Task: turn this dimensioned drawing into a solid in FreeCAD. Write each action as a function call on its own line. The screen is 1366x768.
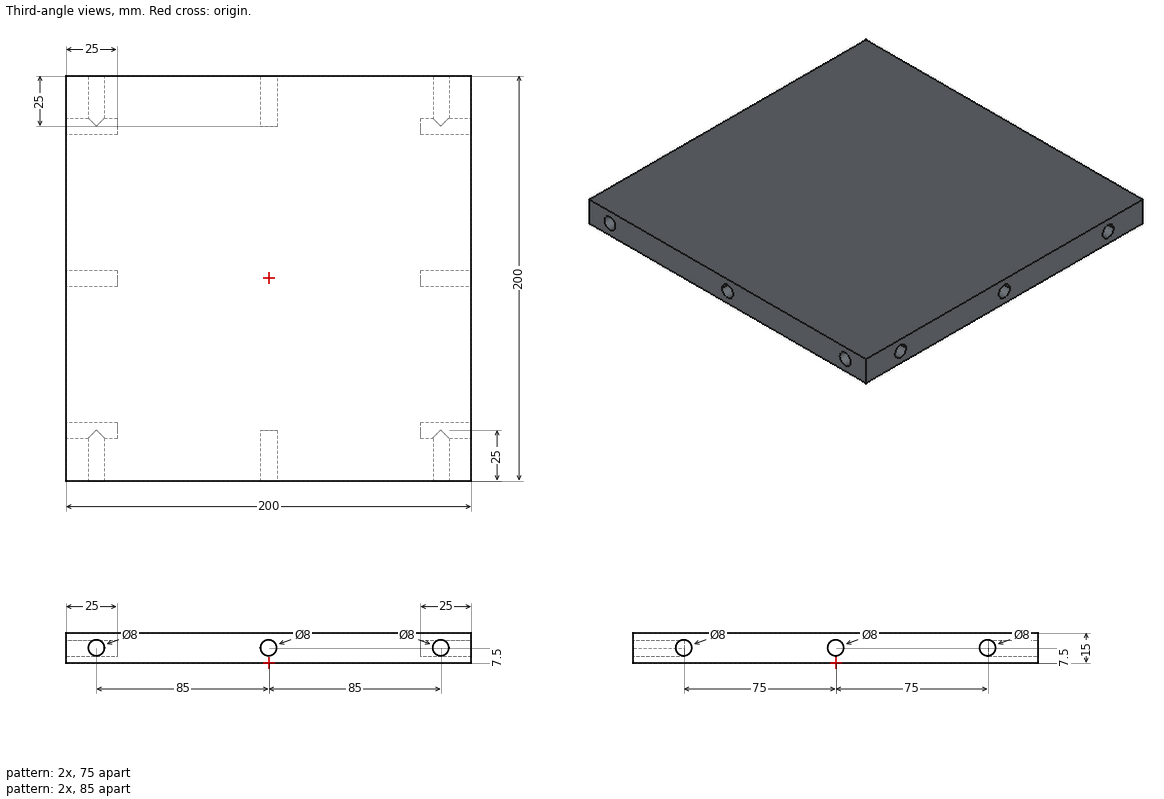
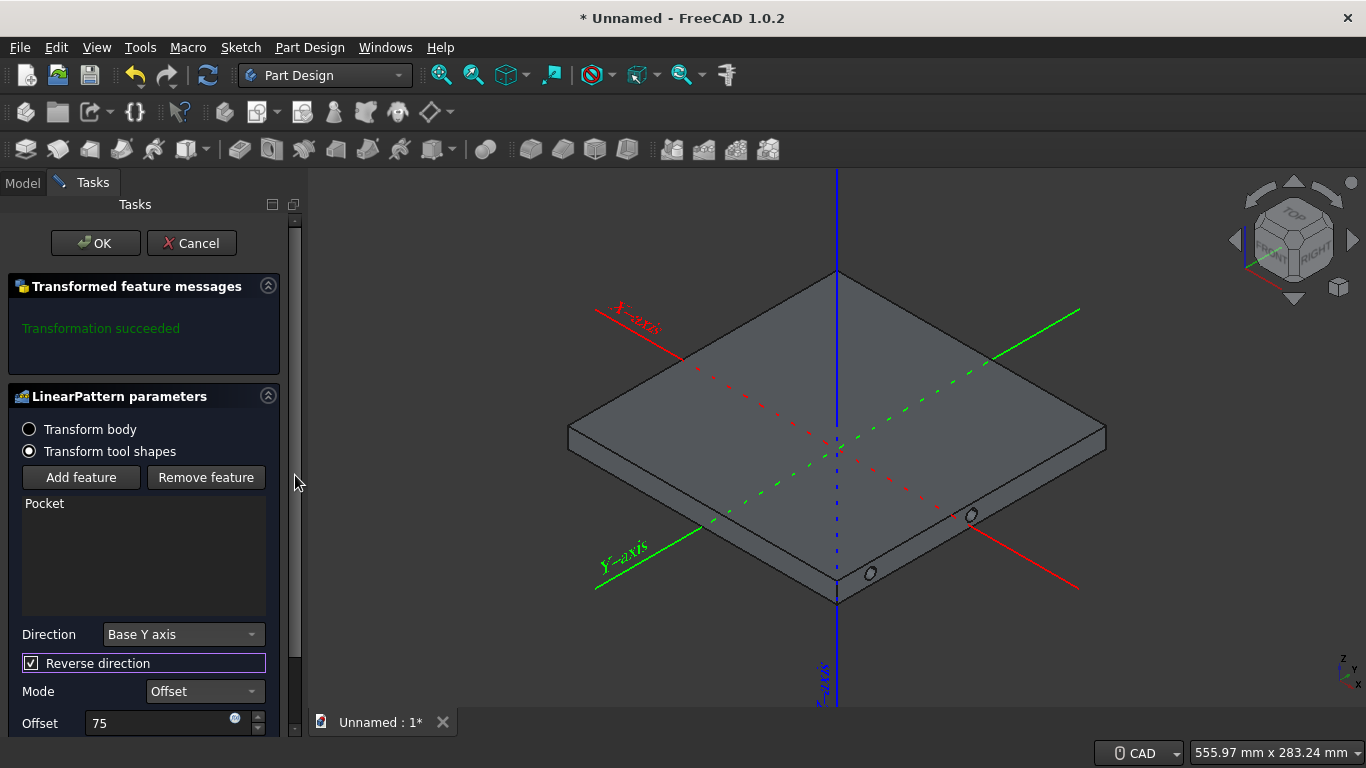
click(96, 243)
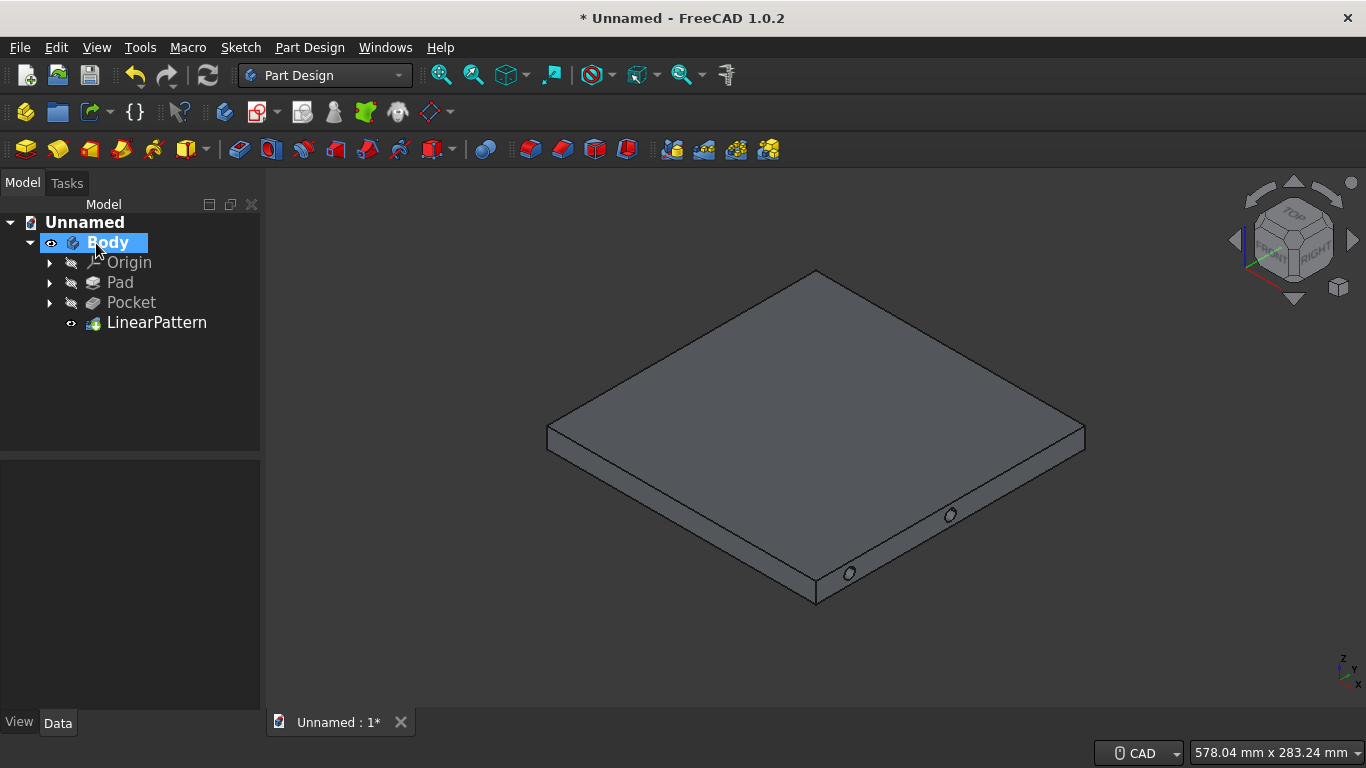
click(1066, 448)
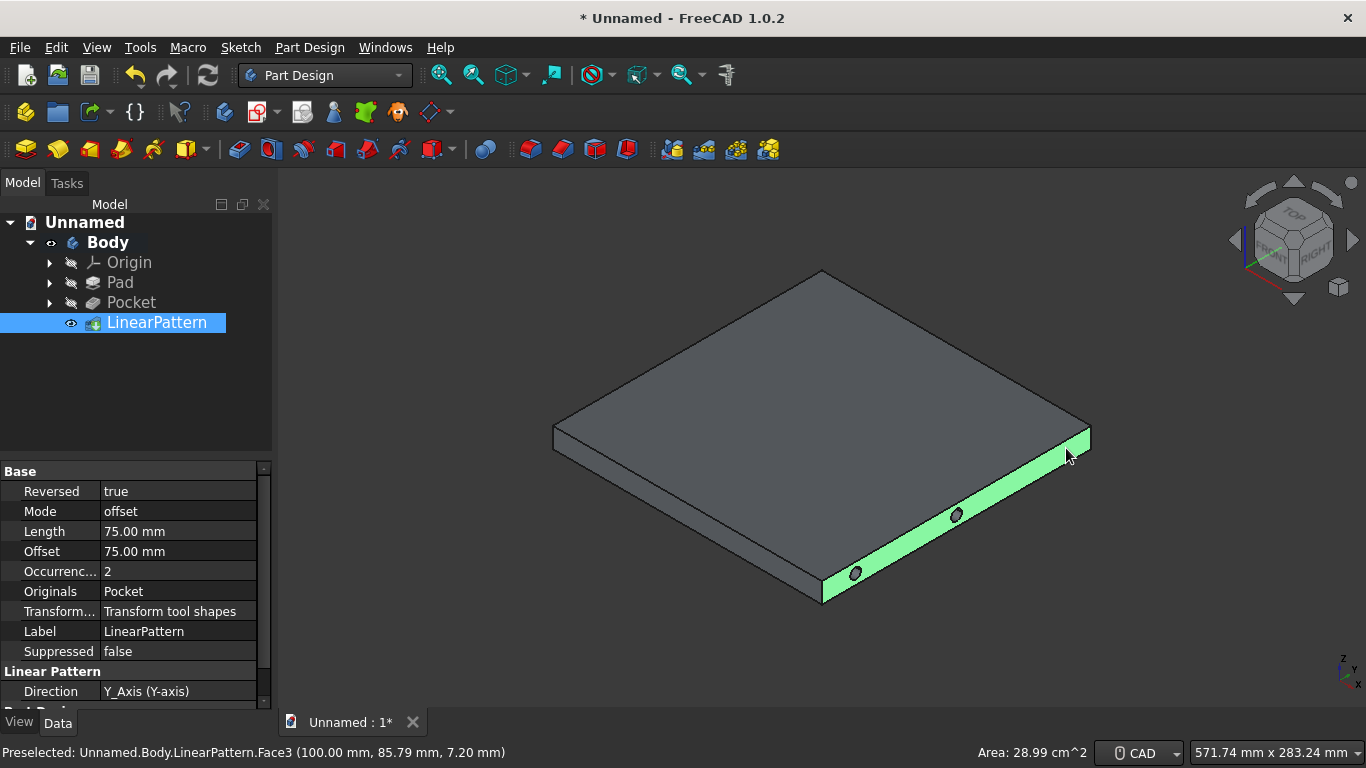
click(258, 112)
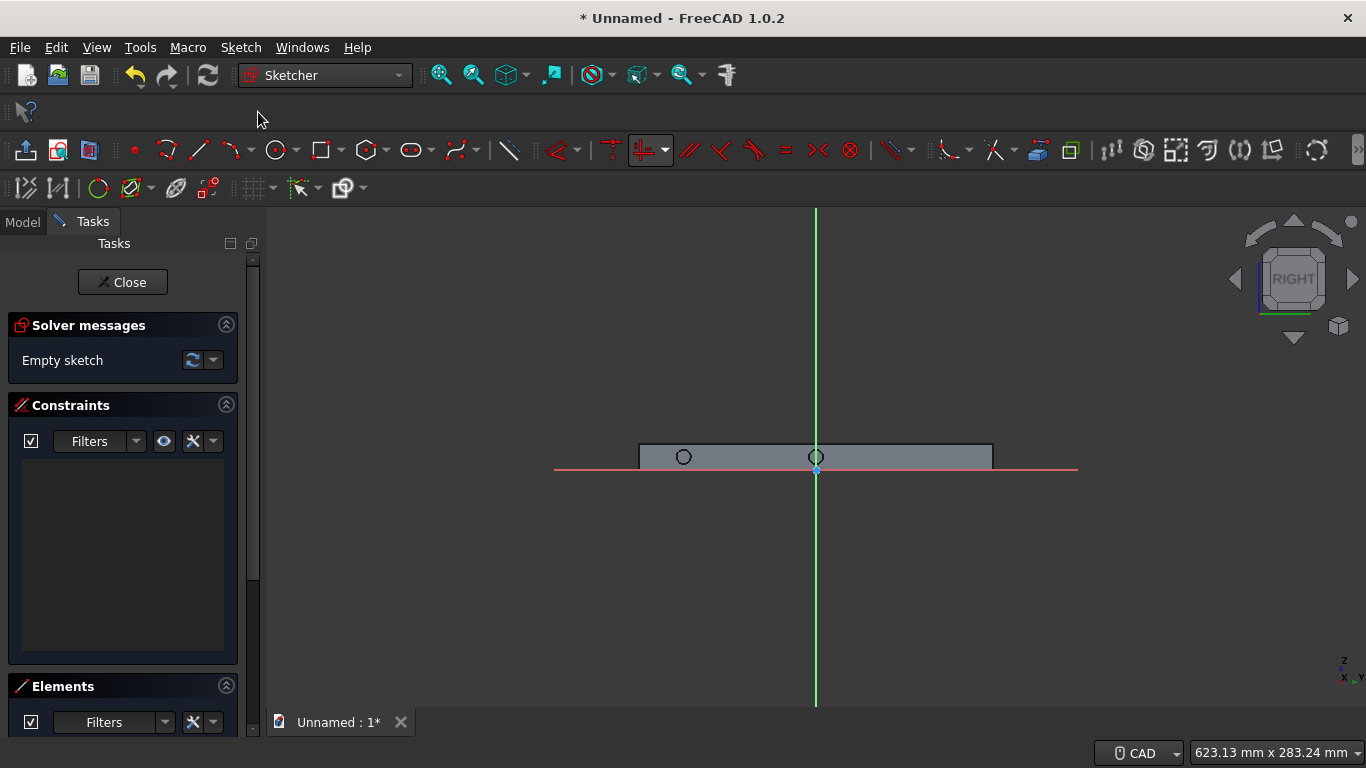
scroll(959, 457, up, 15)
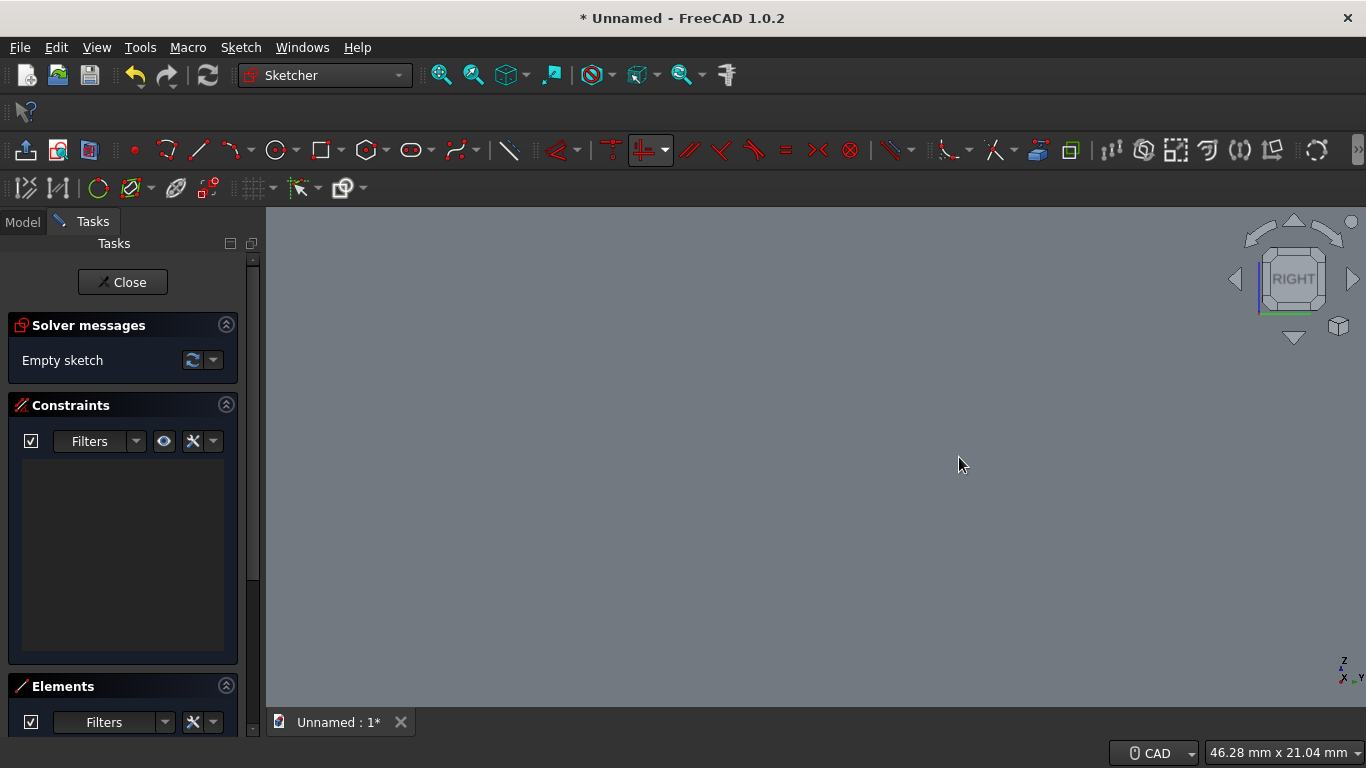
click(276, 150)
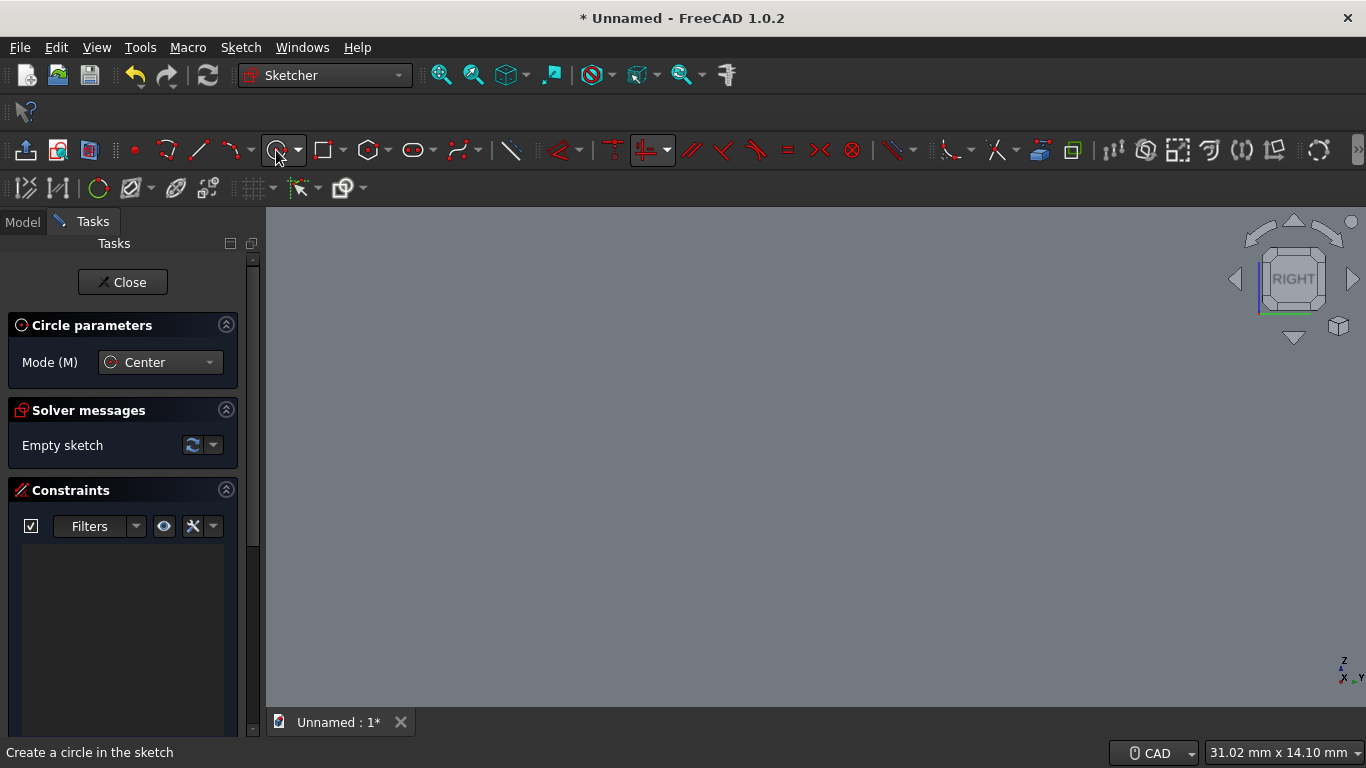
click(734, 447)
move(834, 347)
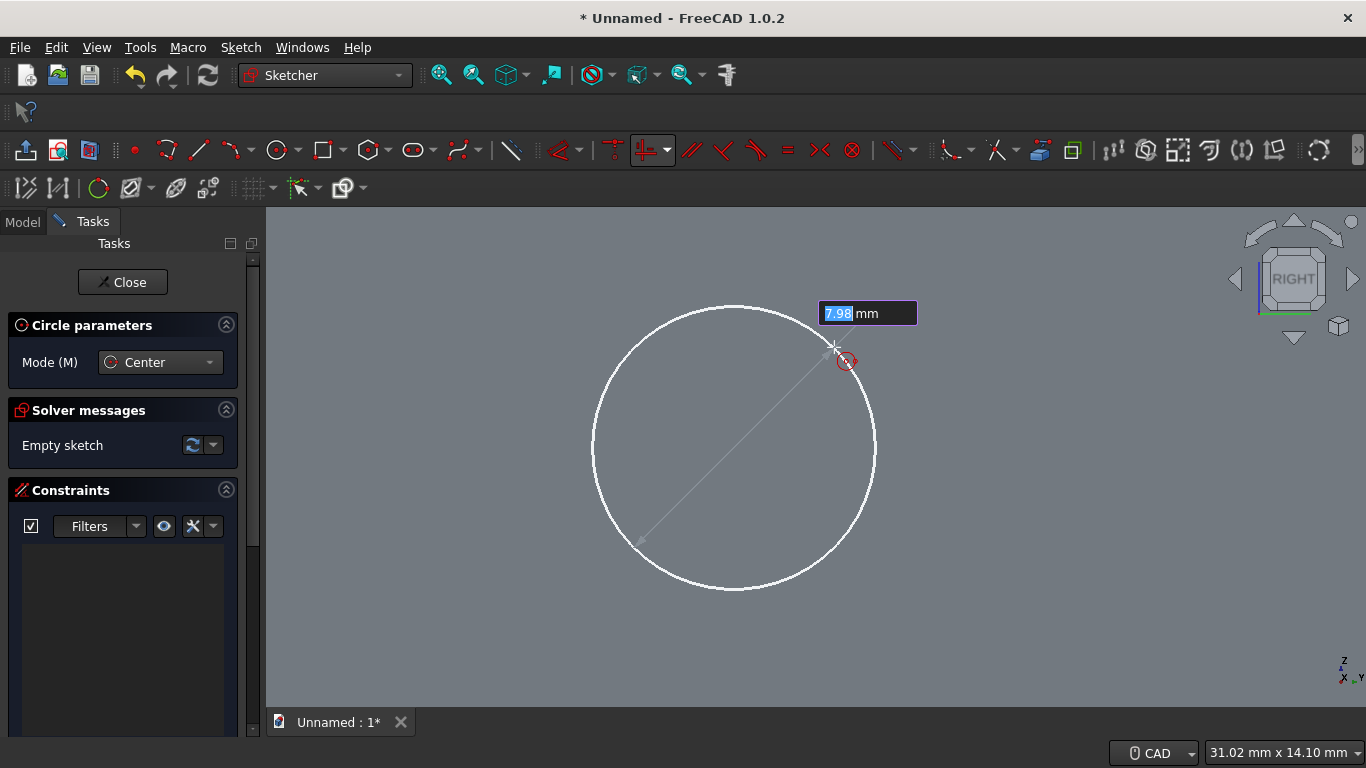
text(8)
key(Return)
key(Escape)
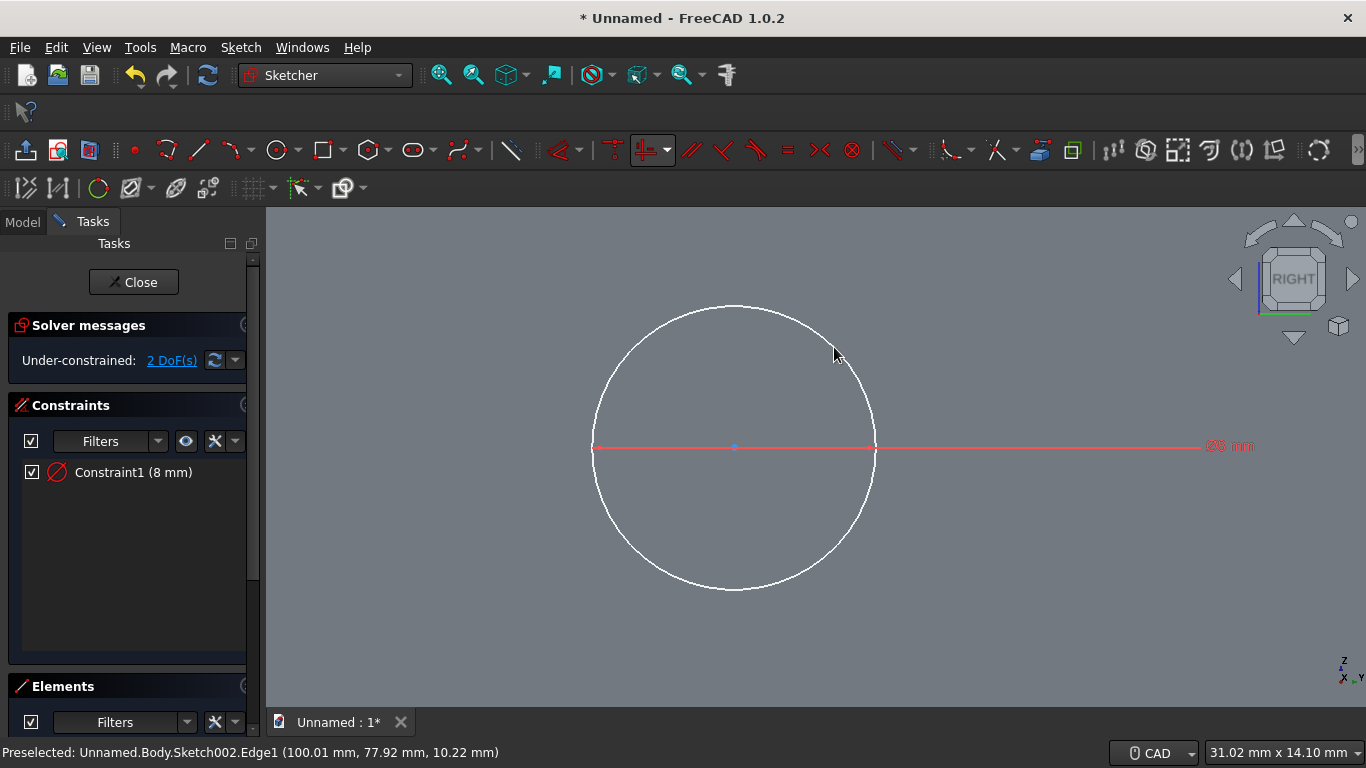
click(558, 150)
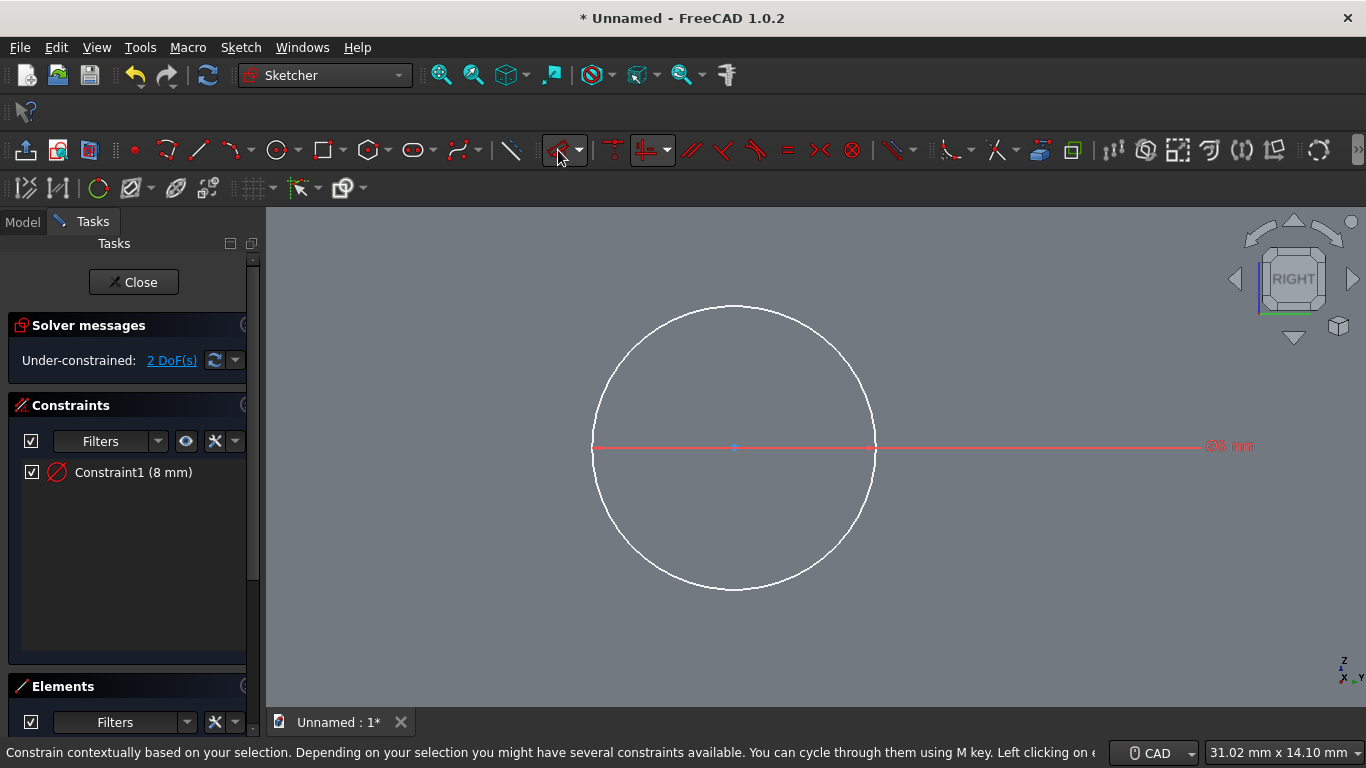
click(734, 448)
click(514, 414)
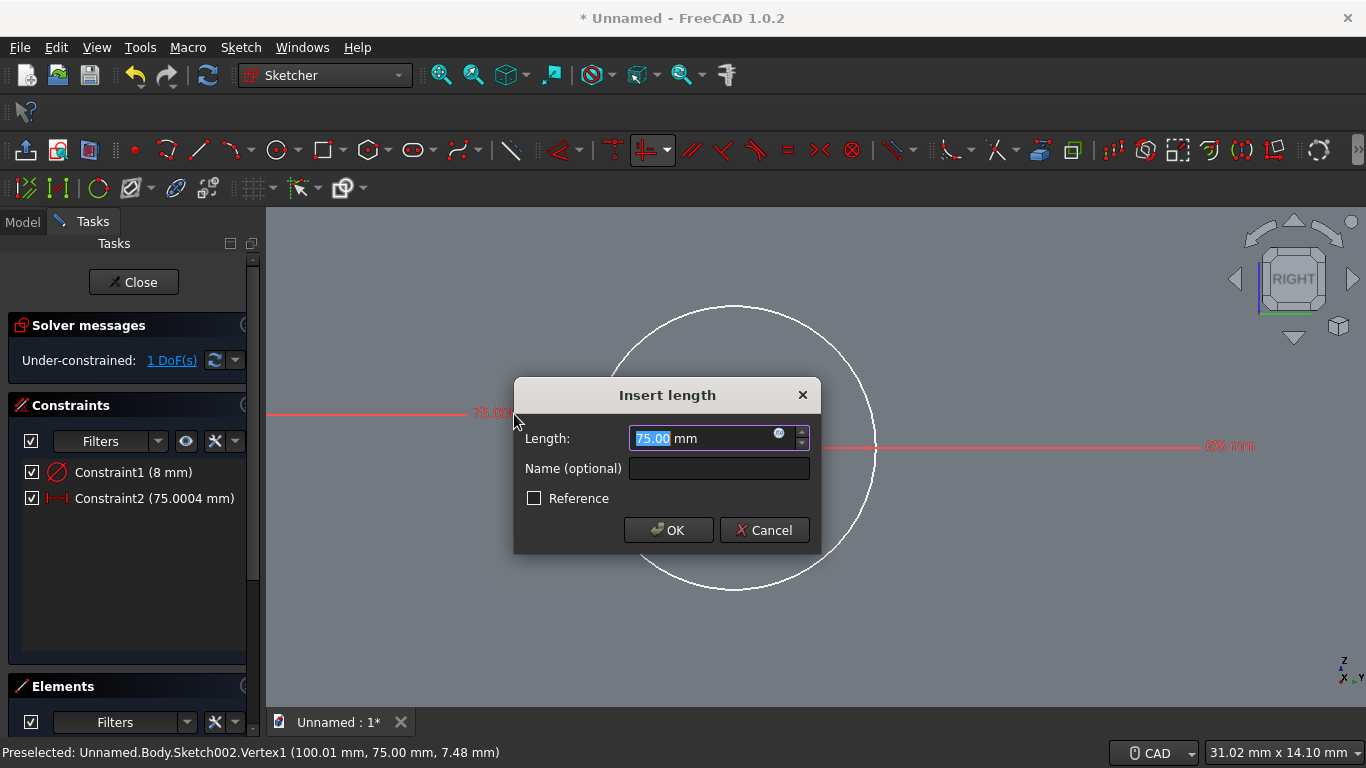
text(75)
key(Return)